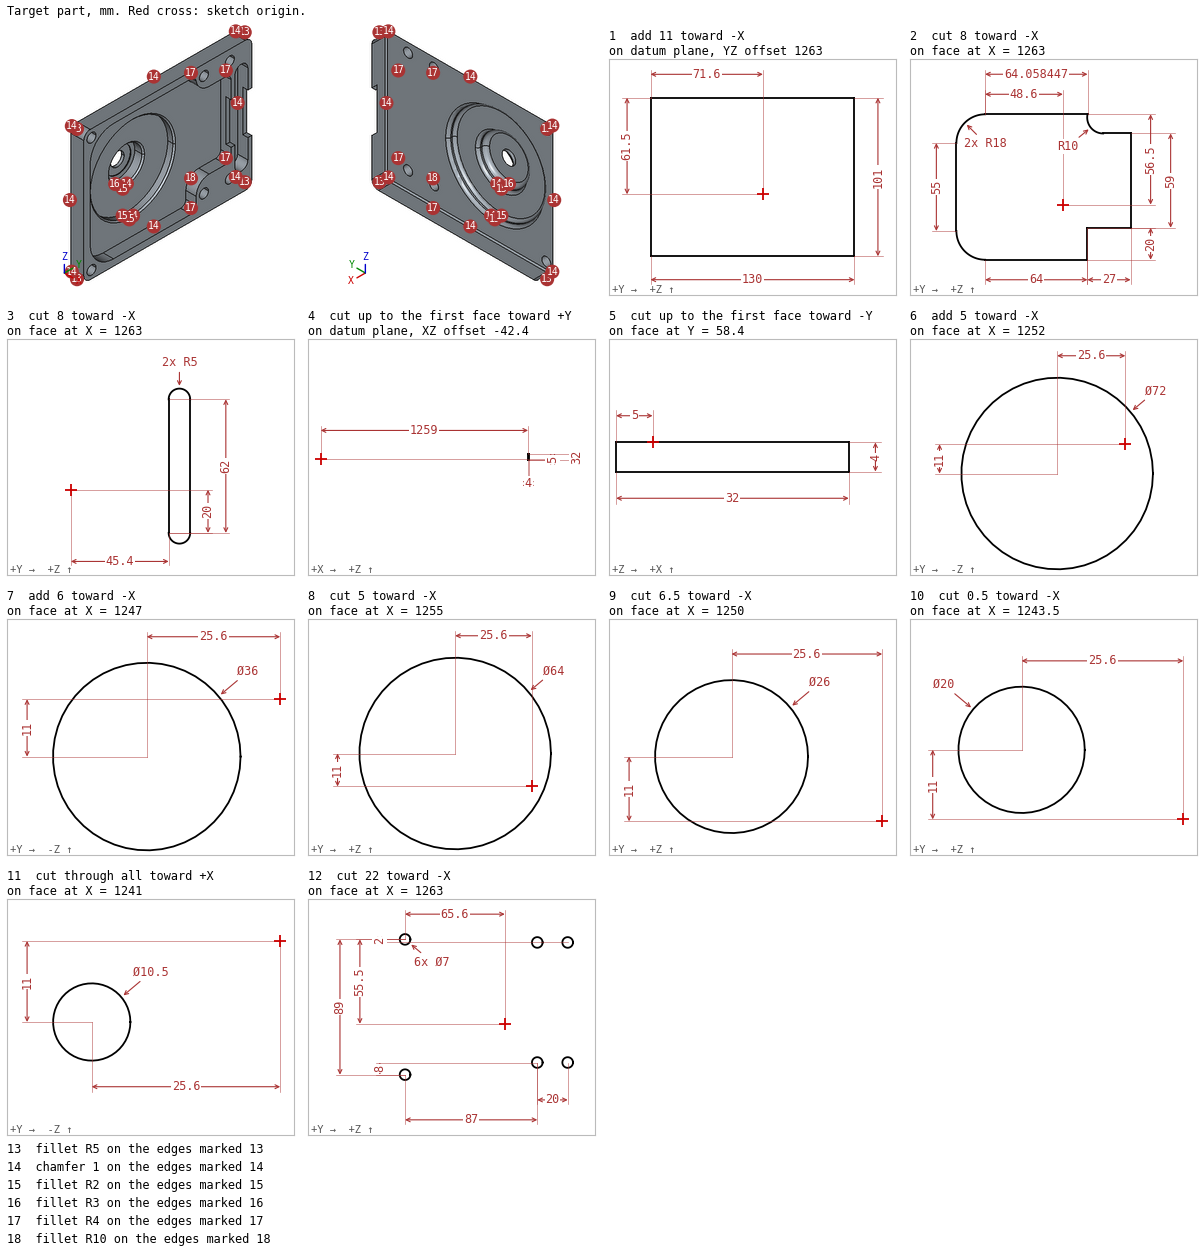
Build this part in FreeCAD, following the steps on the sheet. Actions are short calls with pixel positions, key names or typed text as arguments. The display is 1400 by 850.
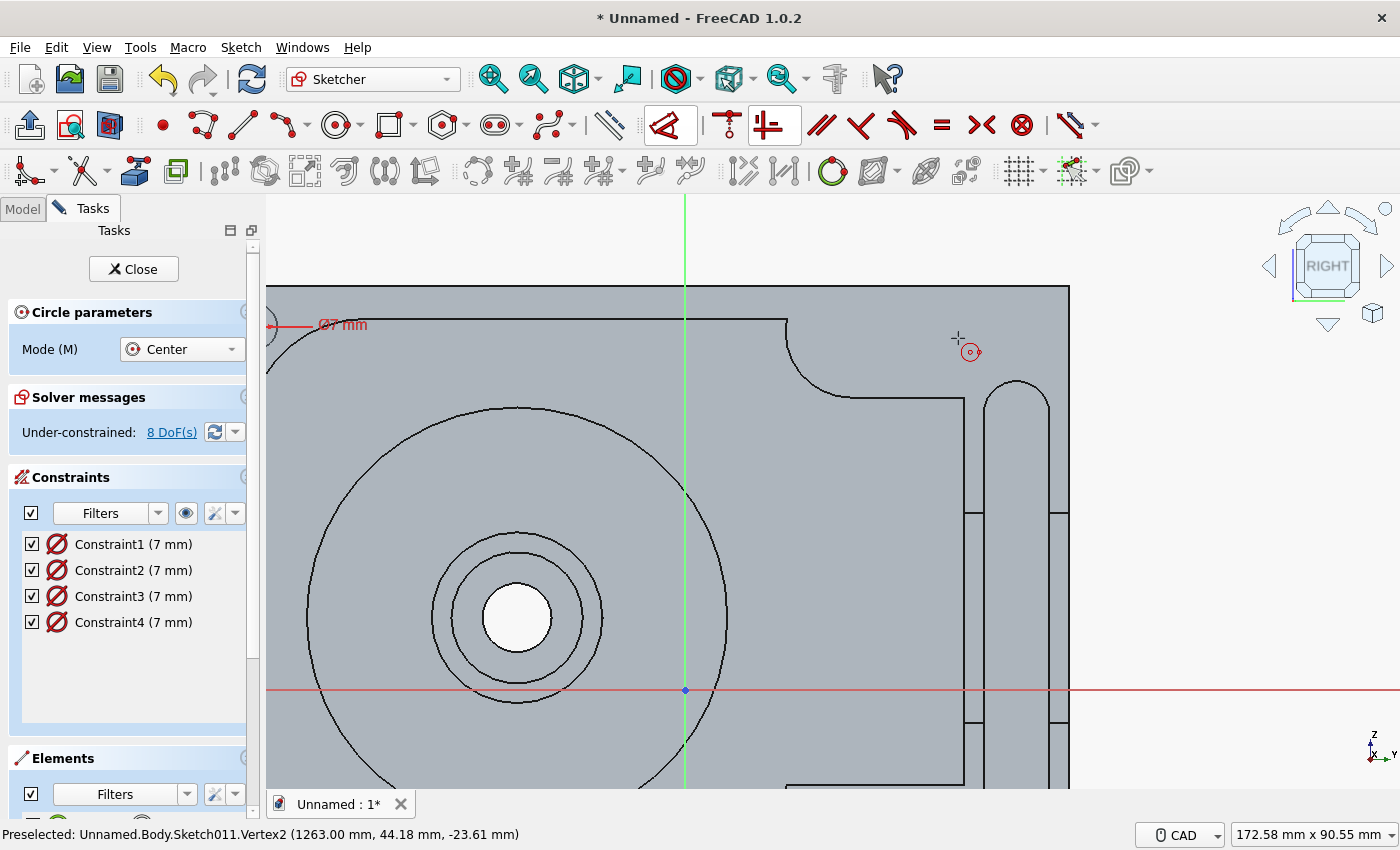
click(957, 338)
move(974, 322)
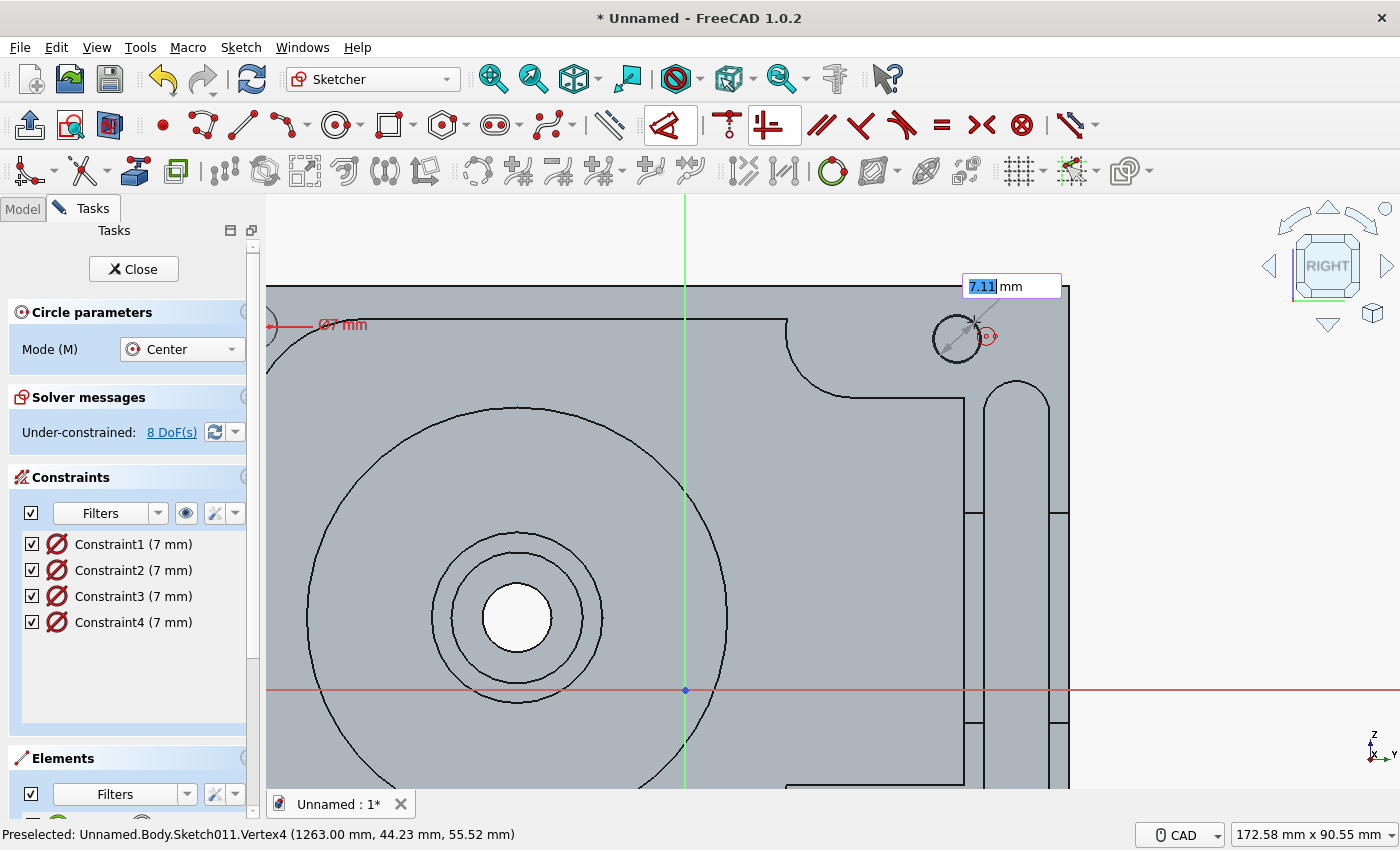
text(7)
key(Return)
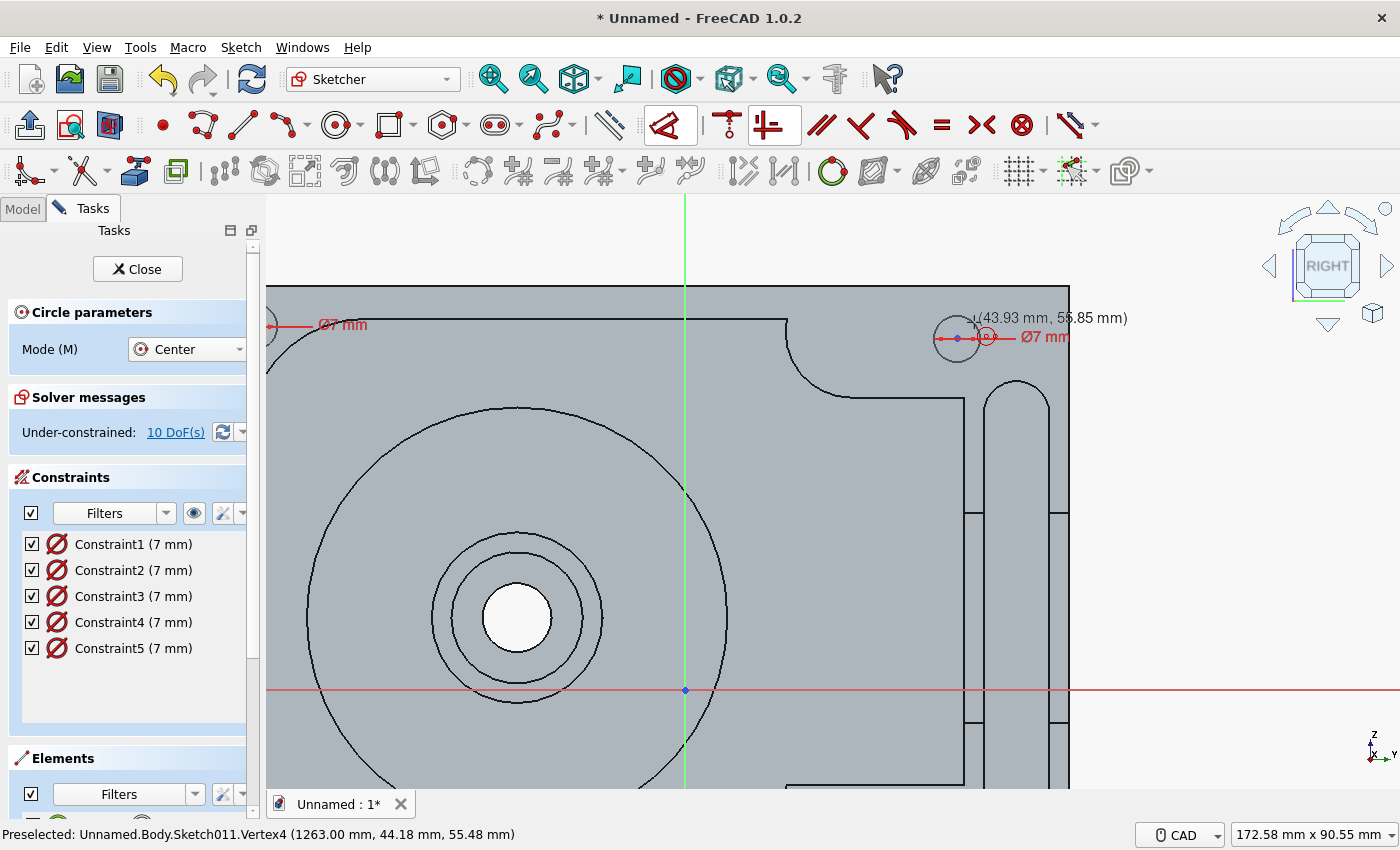
click(826, 338)
move(842, 322)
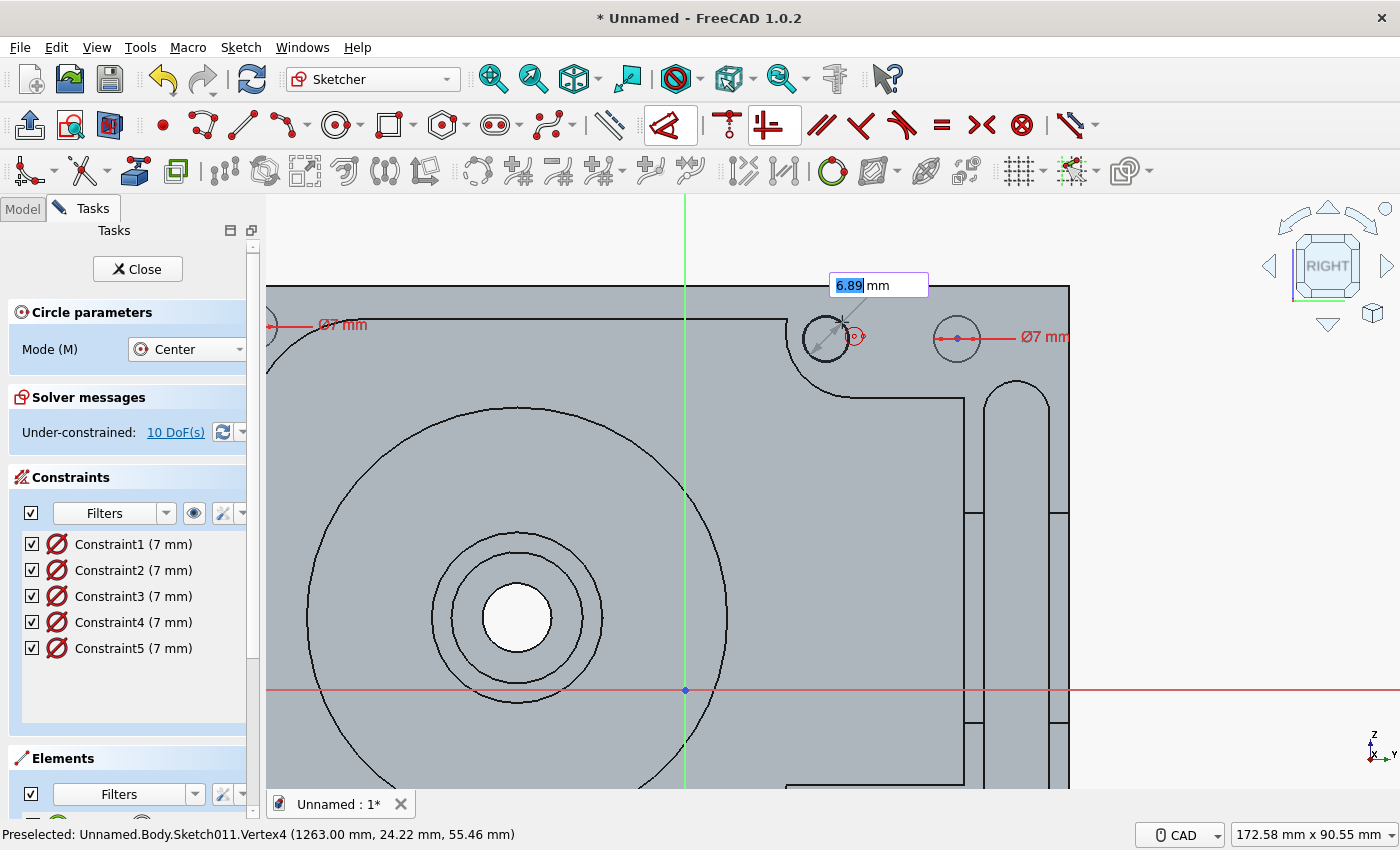
text(7)
key(Return)
key(Escape)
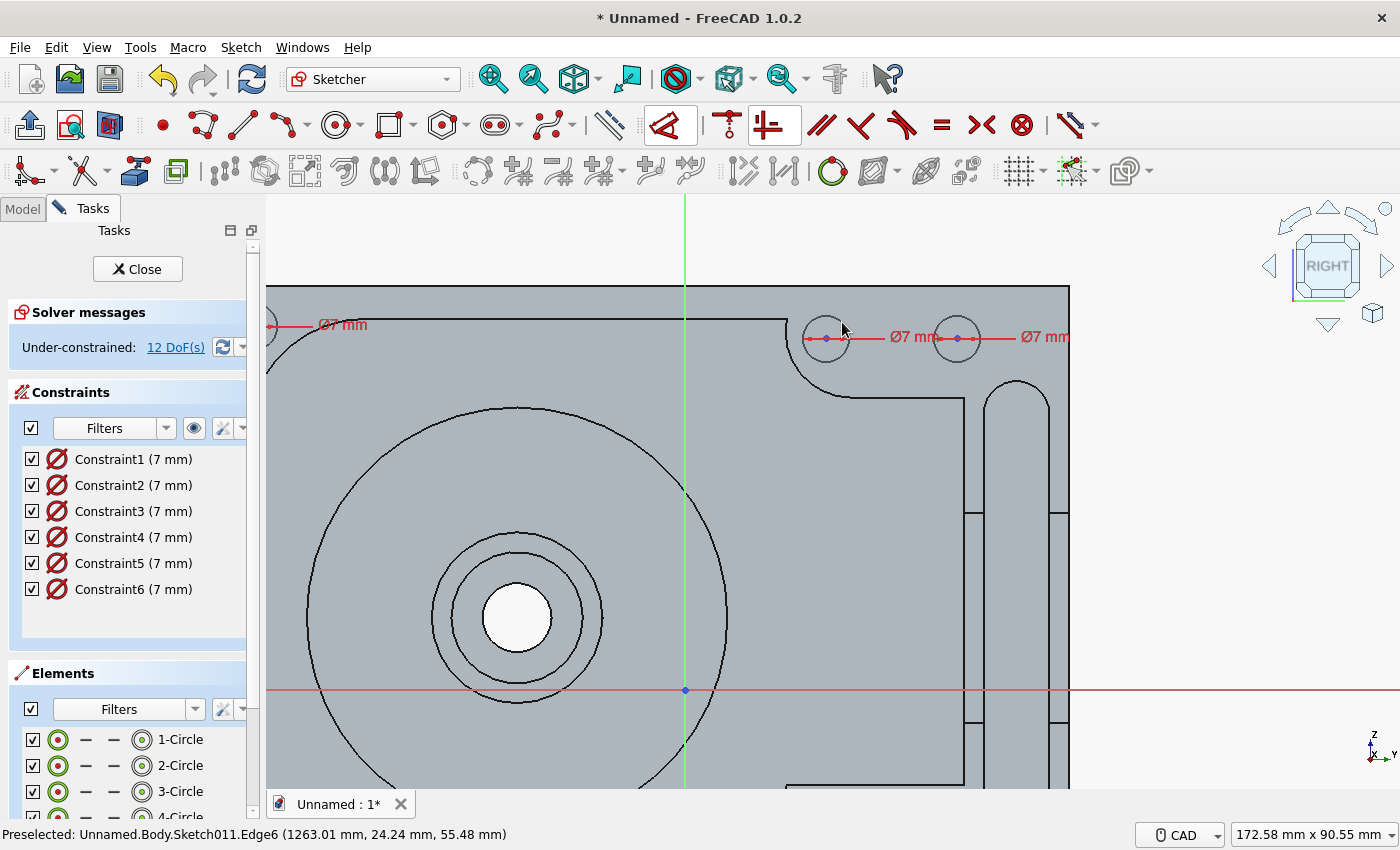
scroll(958, 338, down, 3)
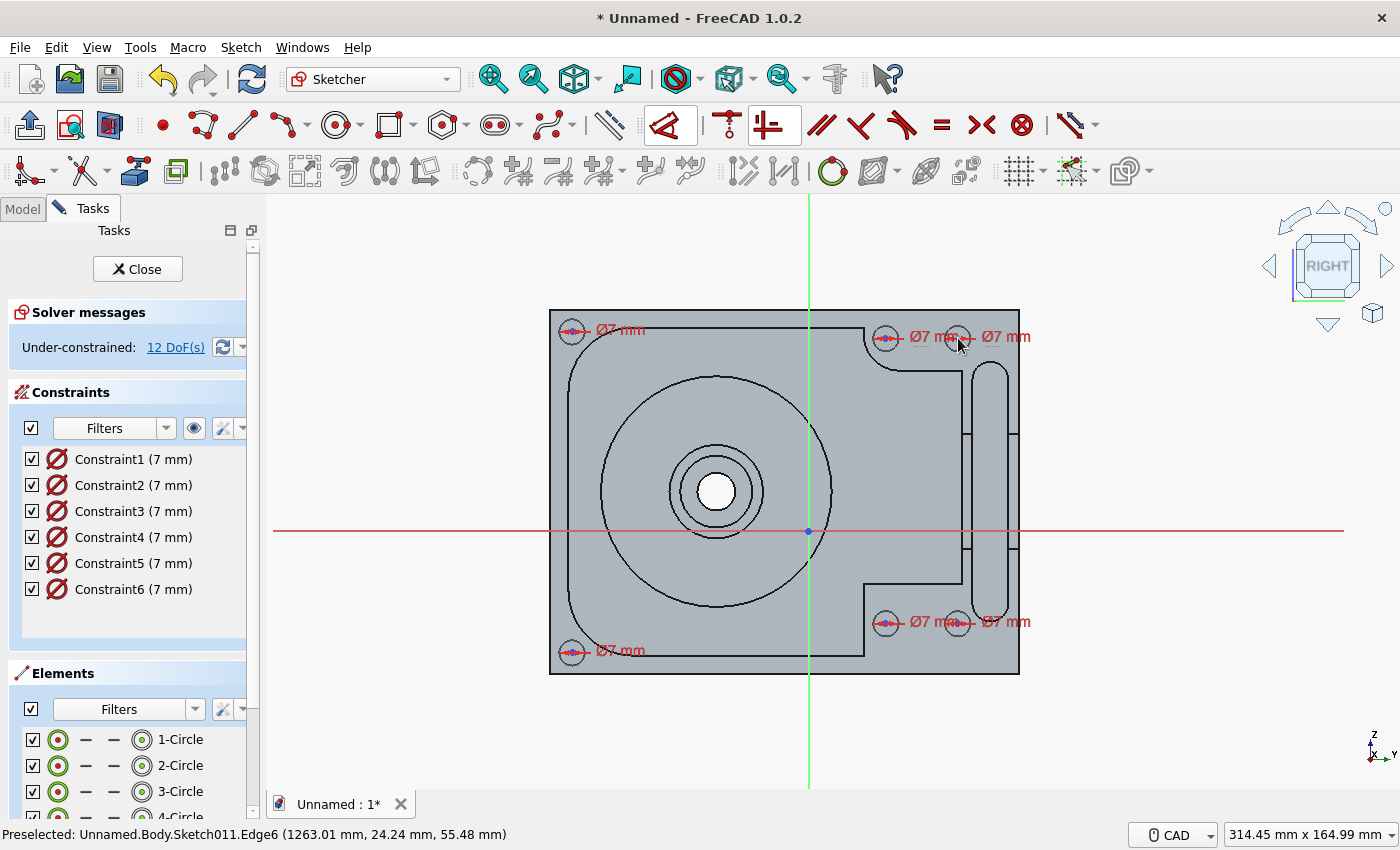
click(572, 332)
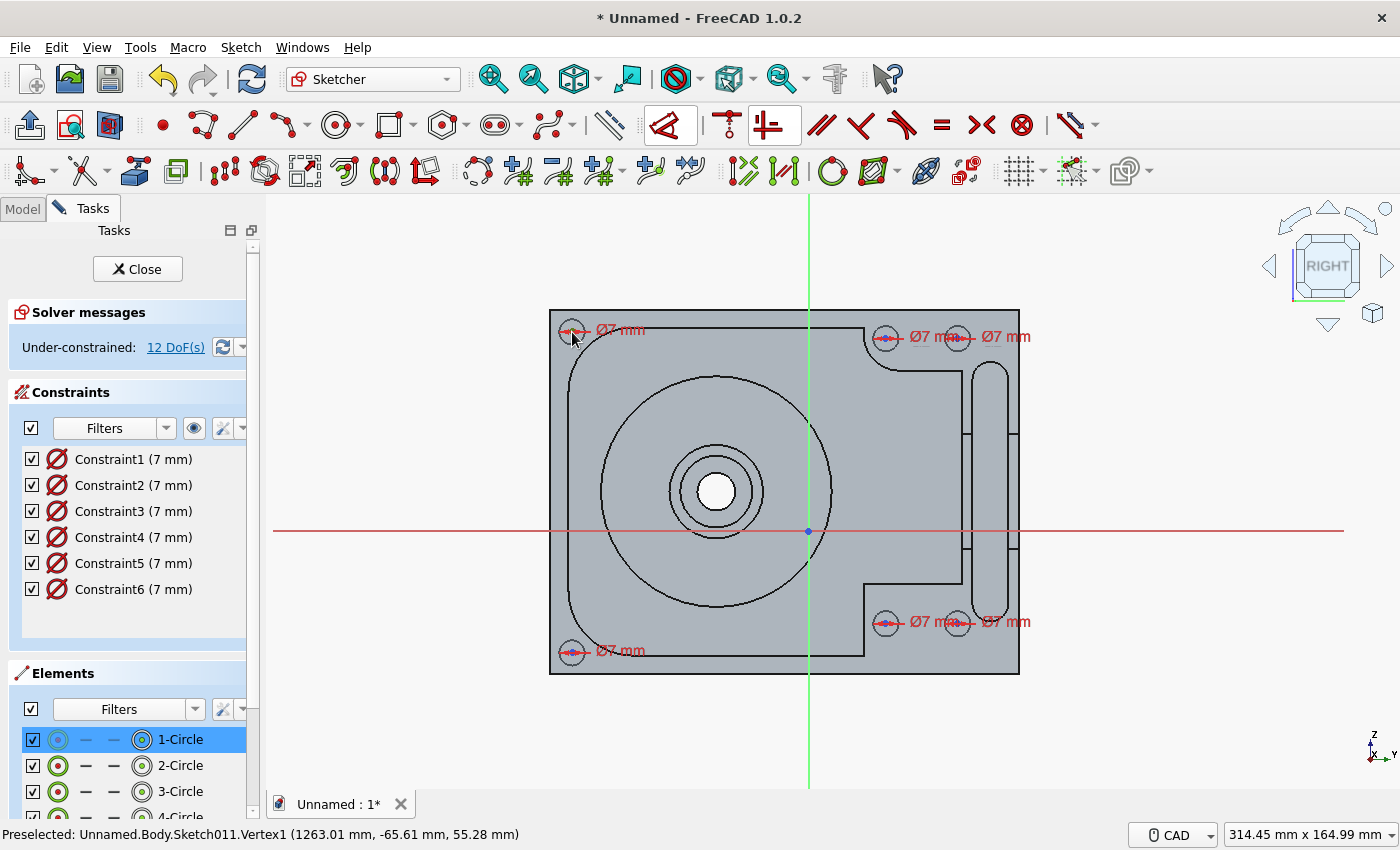
click(572, 653)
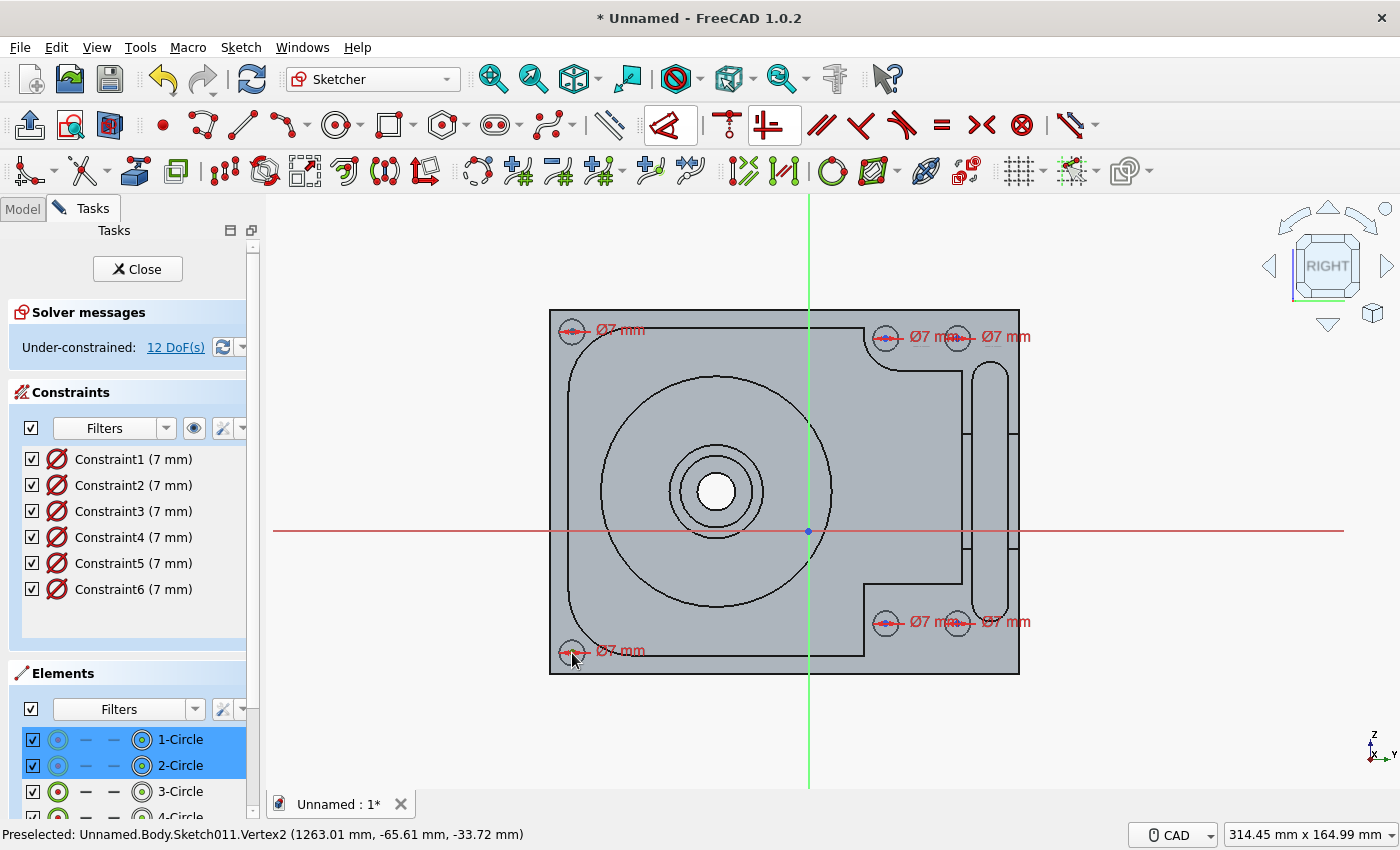
key(v)